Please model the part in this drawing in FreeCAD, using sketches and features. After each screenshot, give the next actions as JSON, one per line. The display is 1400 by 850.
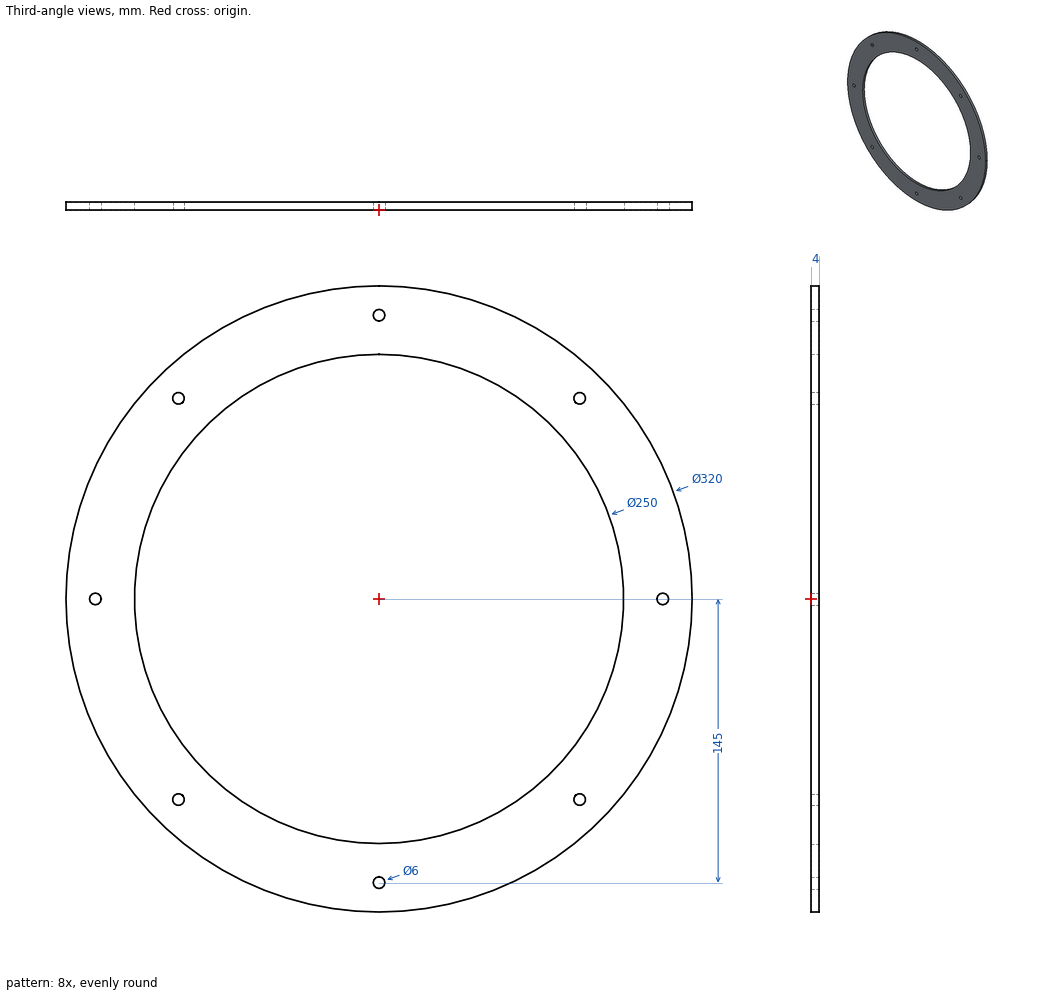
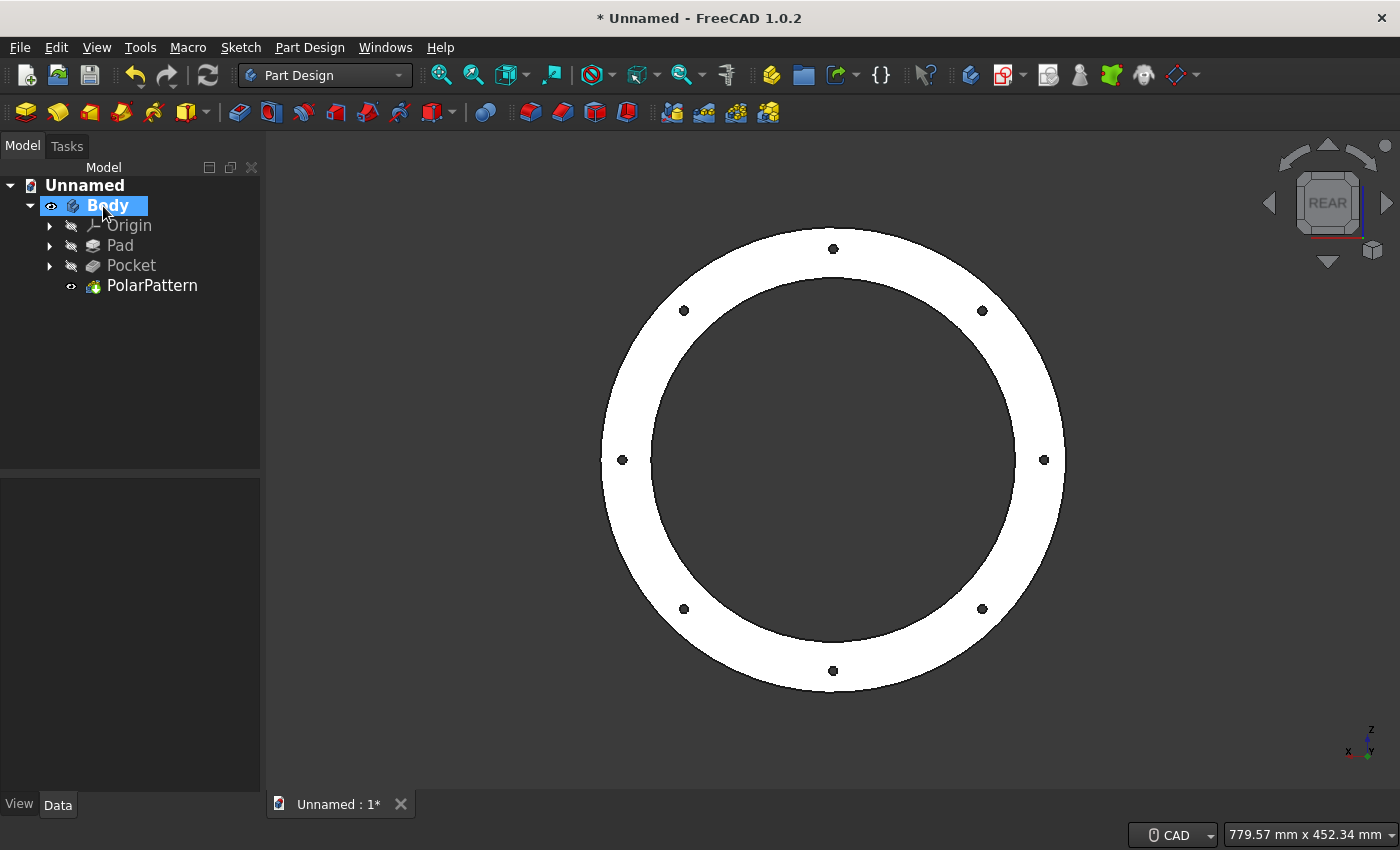
{"action": "key", "text": "0"}